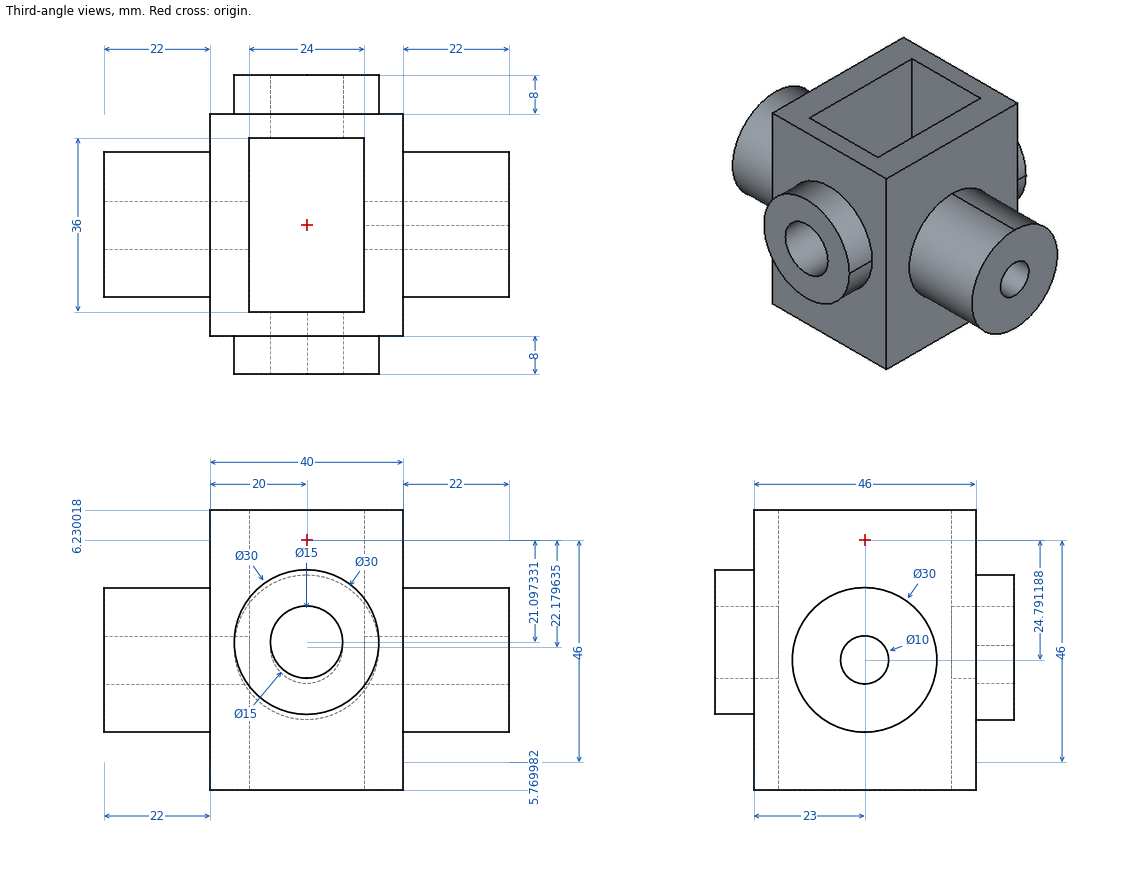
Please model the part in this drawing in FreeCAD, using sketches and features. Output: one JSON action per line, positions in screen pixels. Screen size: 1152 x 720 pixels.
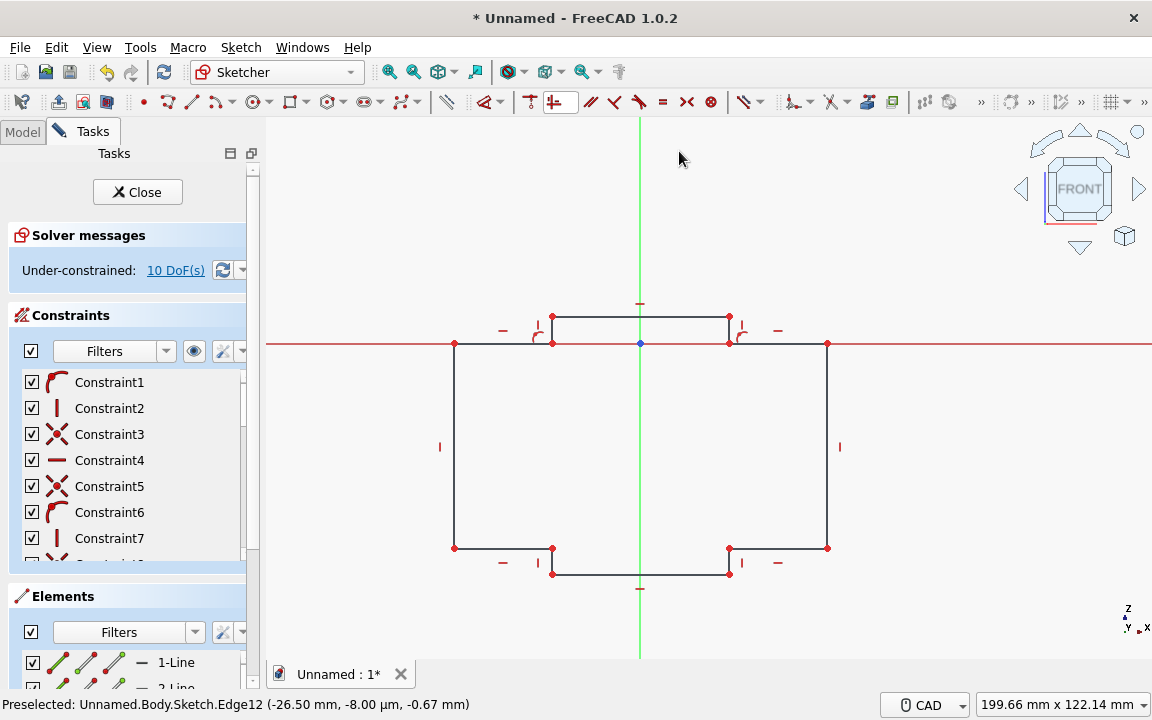
{"action": "left_click", "coordinate": [484, 102]}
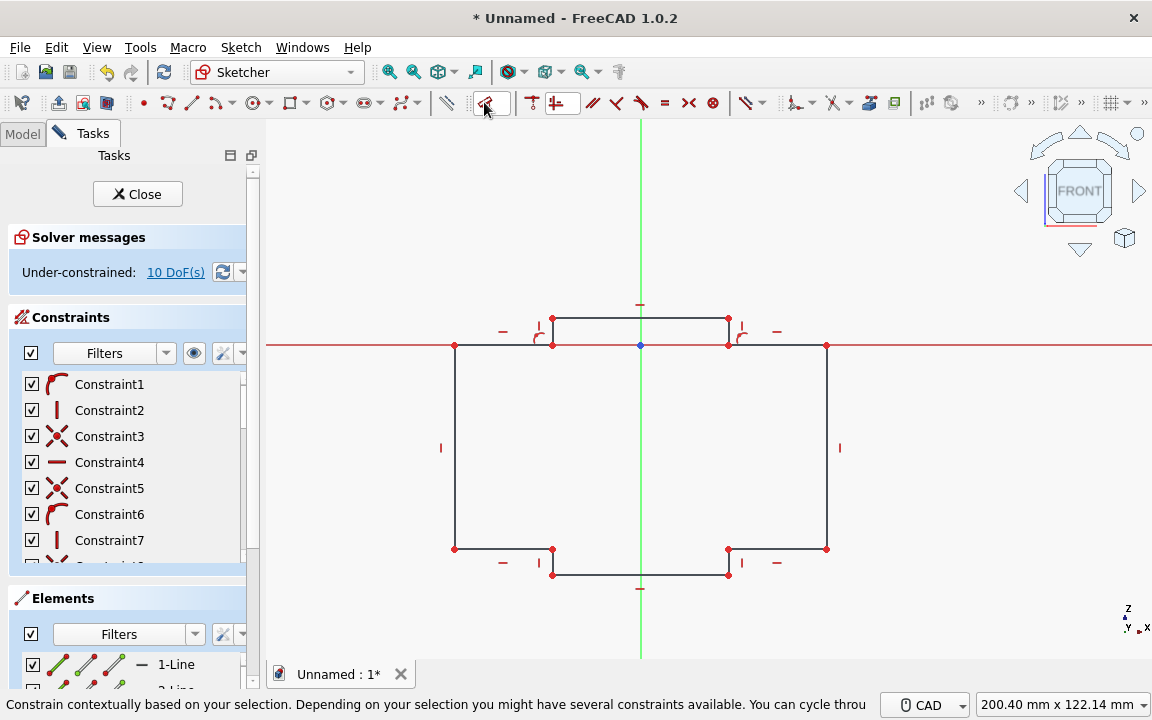
{"action": "left_click", "coordinate": [605, 318]}
{"action": "left_click", "coordinate": [600, 284]}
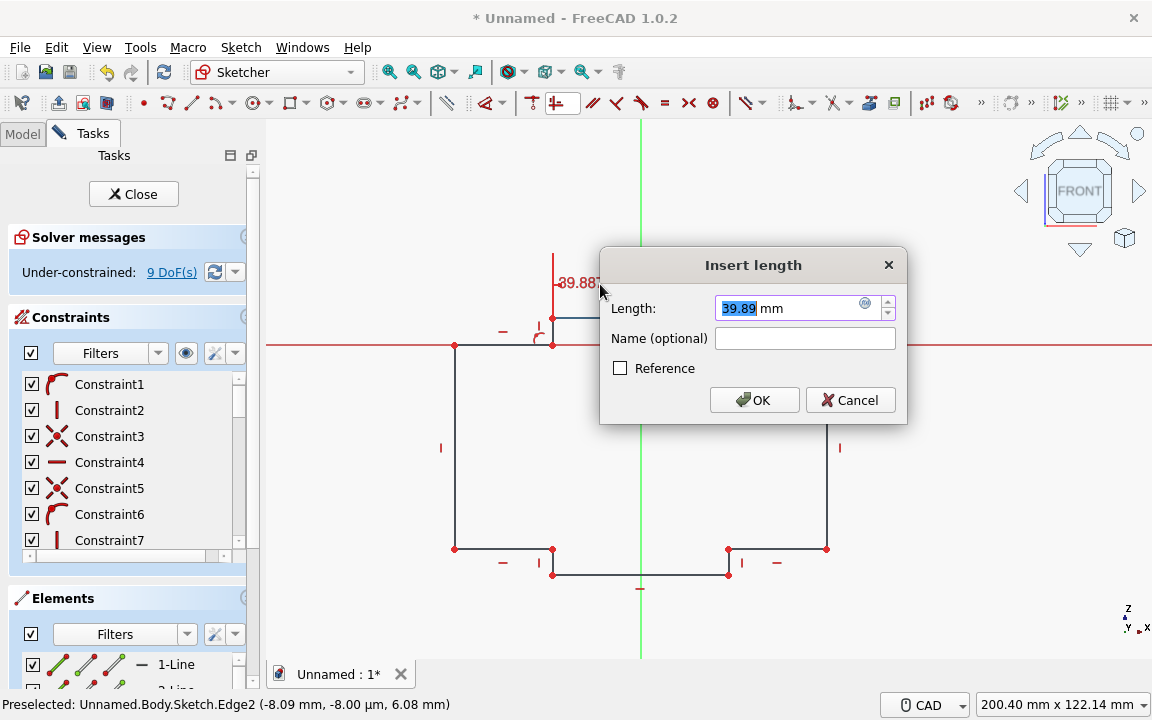
{"action": "type", "text": "40"}
{"action": "key", "text": "Return"}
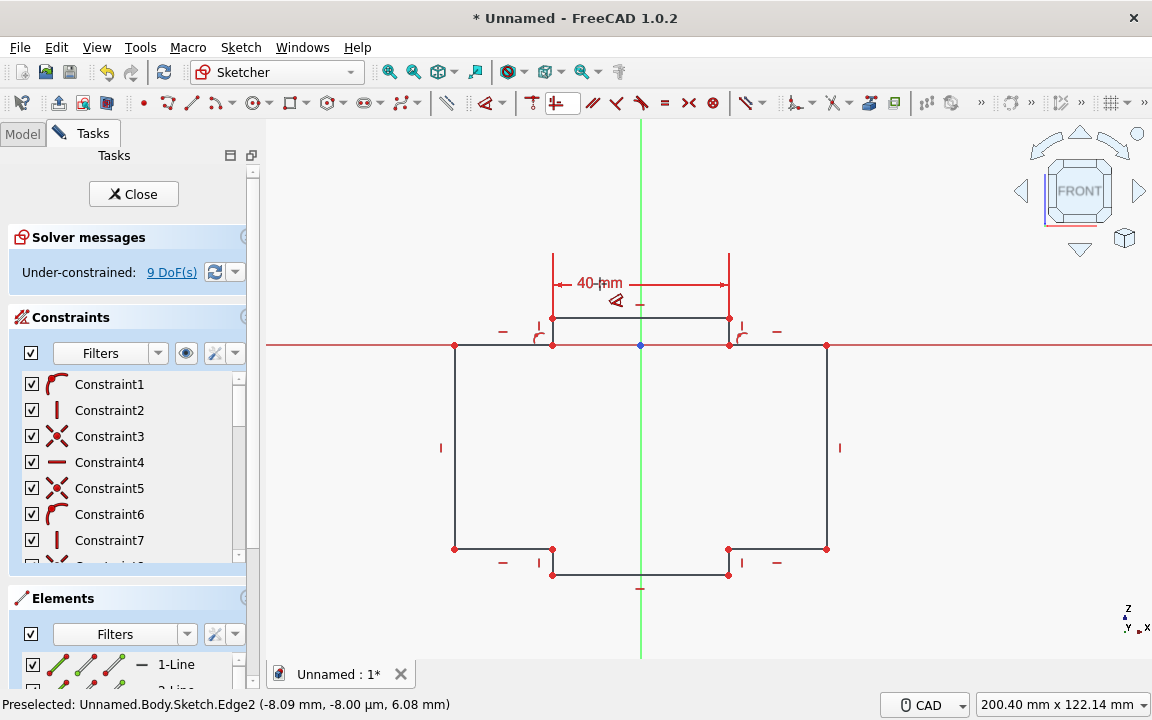
{"action": "left_click", "coordinate": [759, 345]}
{"action": "left_click", "coordinate": [778, 311]}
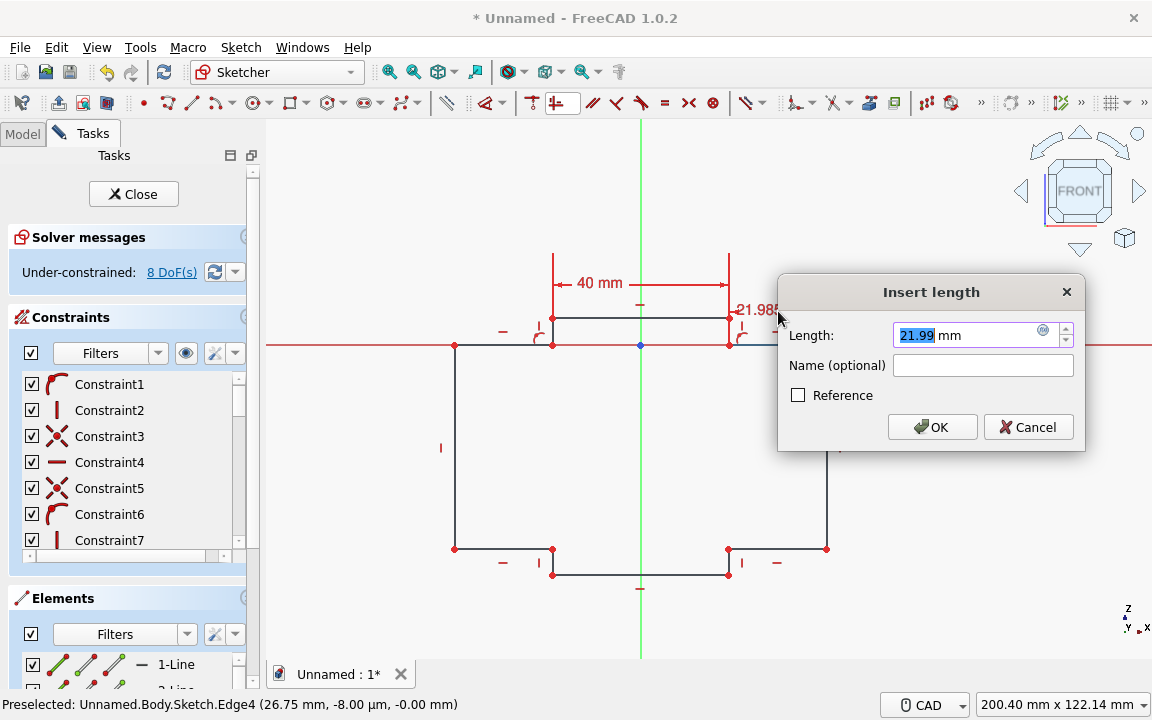
{"action": "type", "text": "22"}
{"action": "key", "text": "Return"}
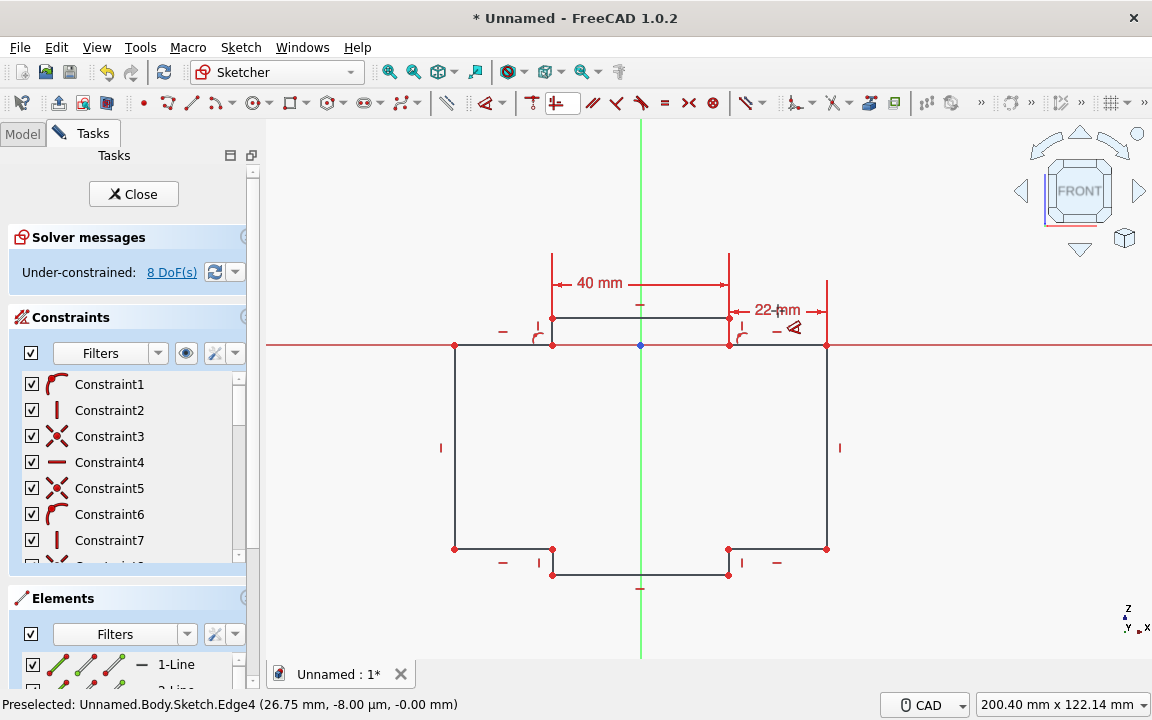
{"action": "left_click", "coordinate": [827, 406]}
{"action": "left_click", "coordinate": [861, 447]}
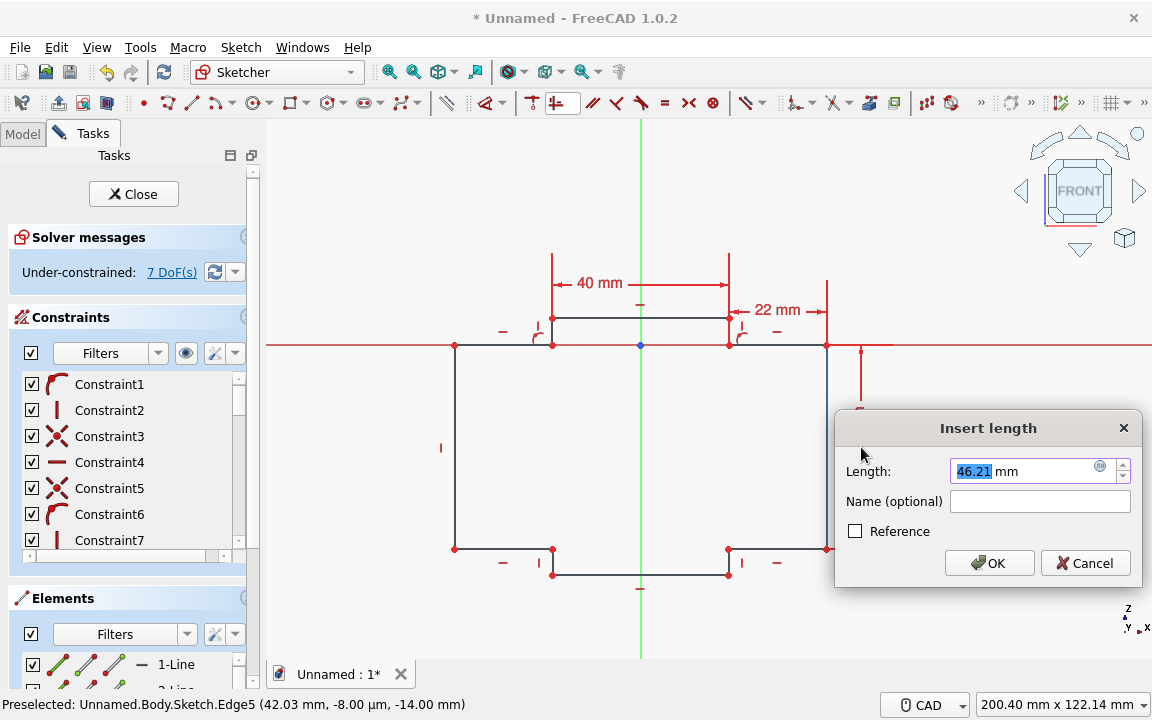
{"action": "type", "text": "46"}
{"action": "key", "text": "Return"}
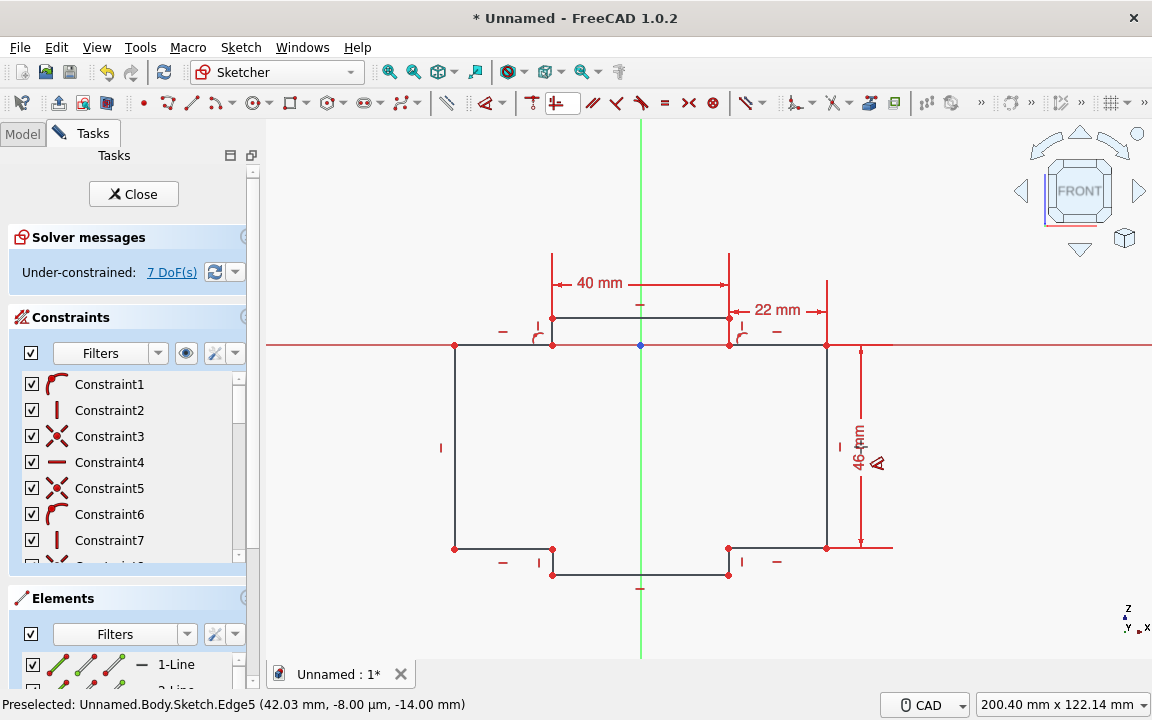
{"action": "left_click", "coordinate": [797, 548]}
{"action": "left_click", "coordinate": [778, 582]}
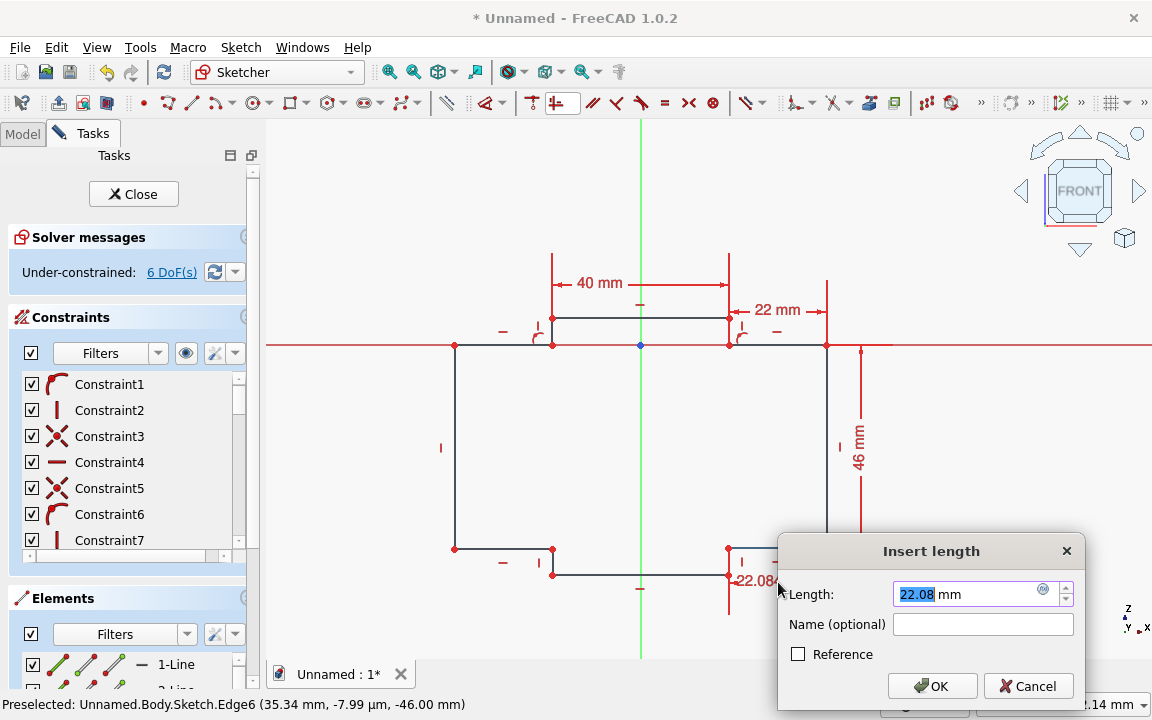
{"action": "type", "text": "22"}
{"action": "key", "text": "Return"}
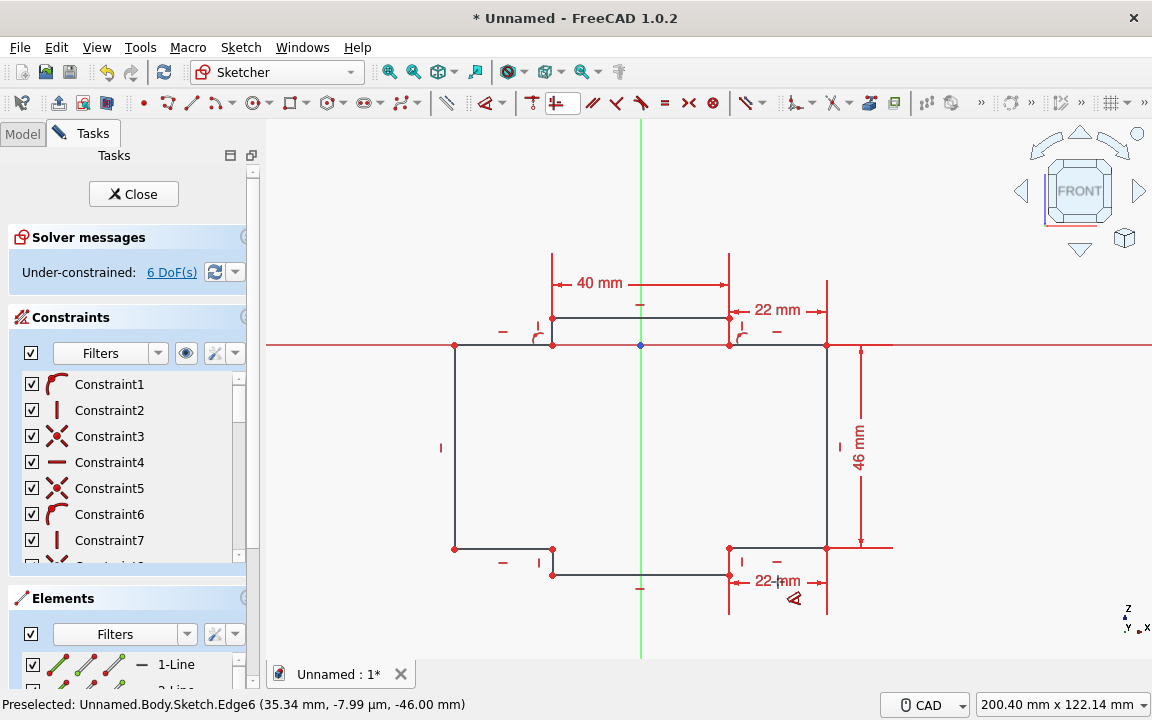
{"action": "left_click", "coordinate": [676, 575]}
{"action": "left_click", "coordinate": [600, 609]}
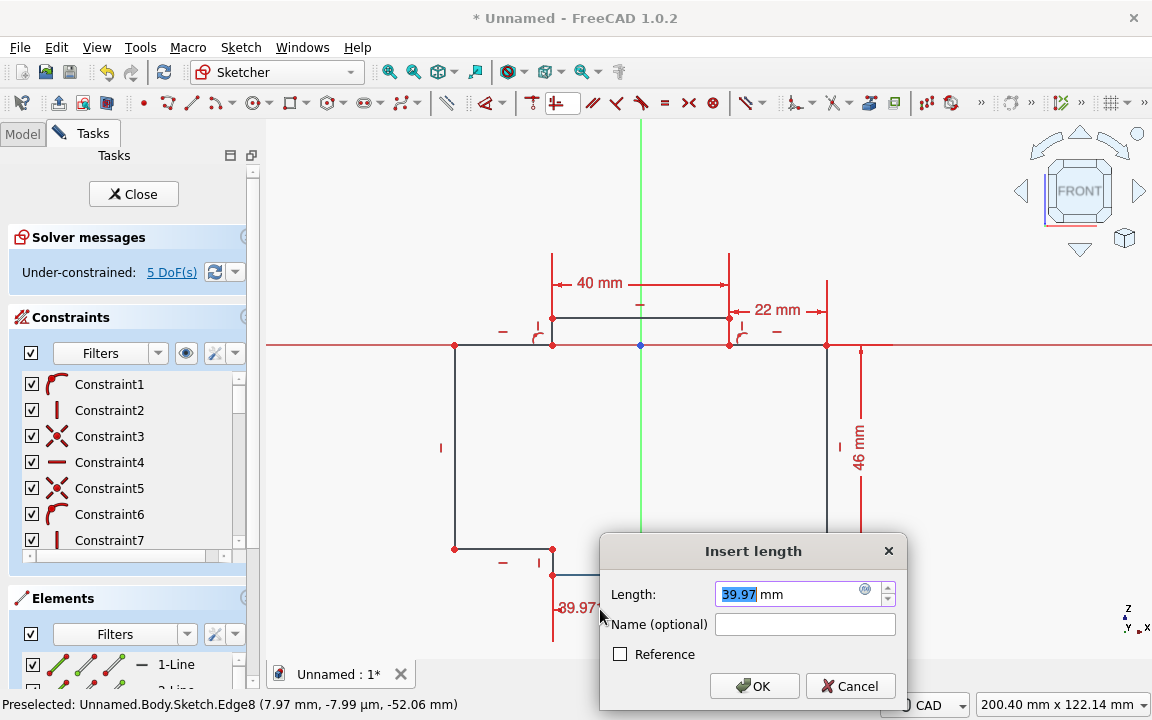
{"action": "type", "text": "40"}
{"action": "key", "text": "Return"}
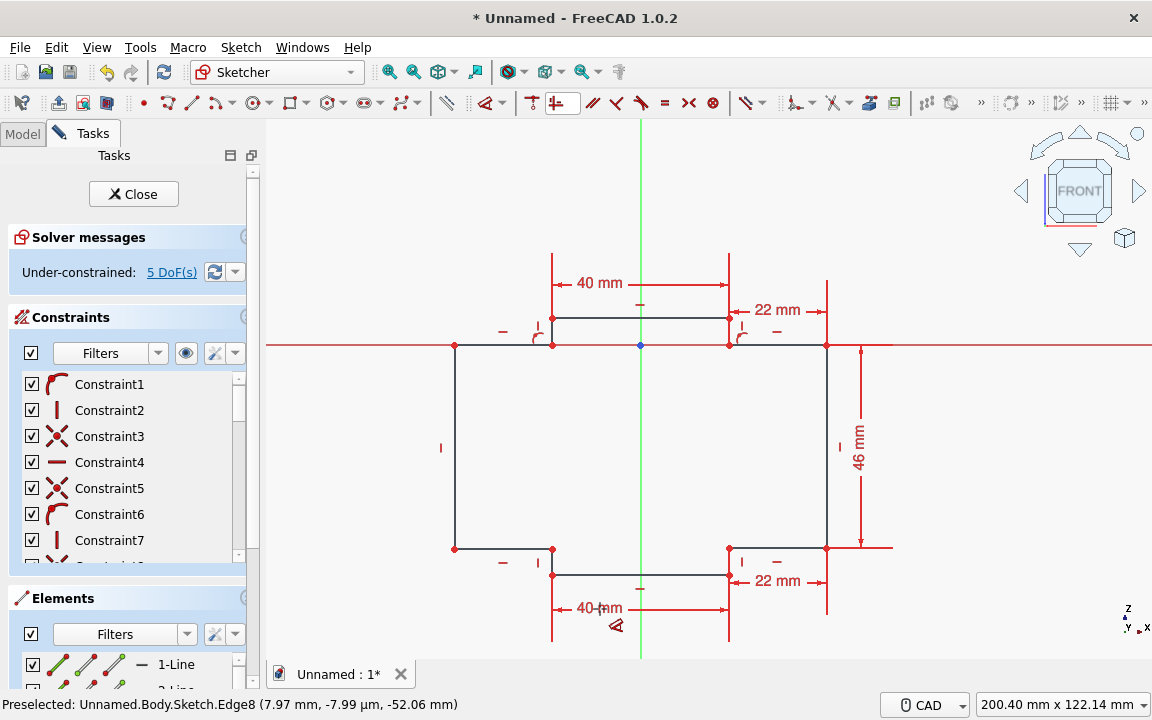
{"action": "left_click", "coordinate": [523, 549]}
{"action": "left_click", "coordinate": [504, 583]}